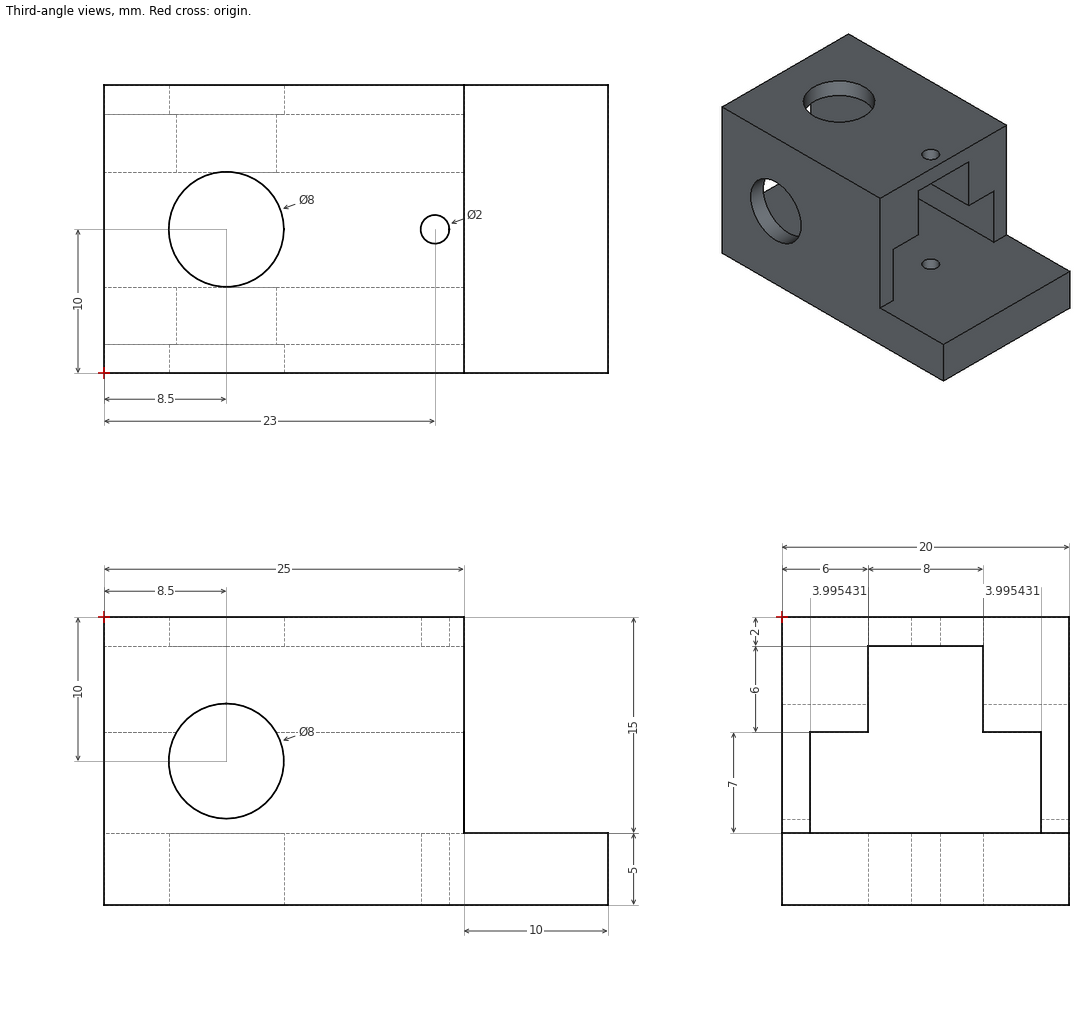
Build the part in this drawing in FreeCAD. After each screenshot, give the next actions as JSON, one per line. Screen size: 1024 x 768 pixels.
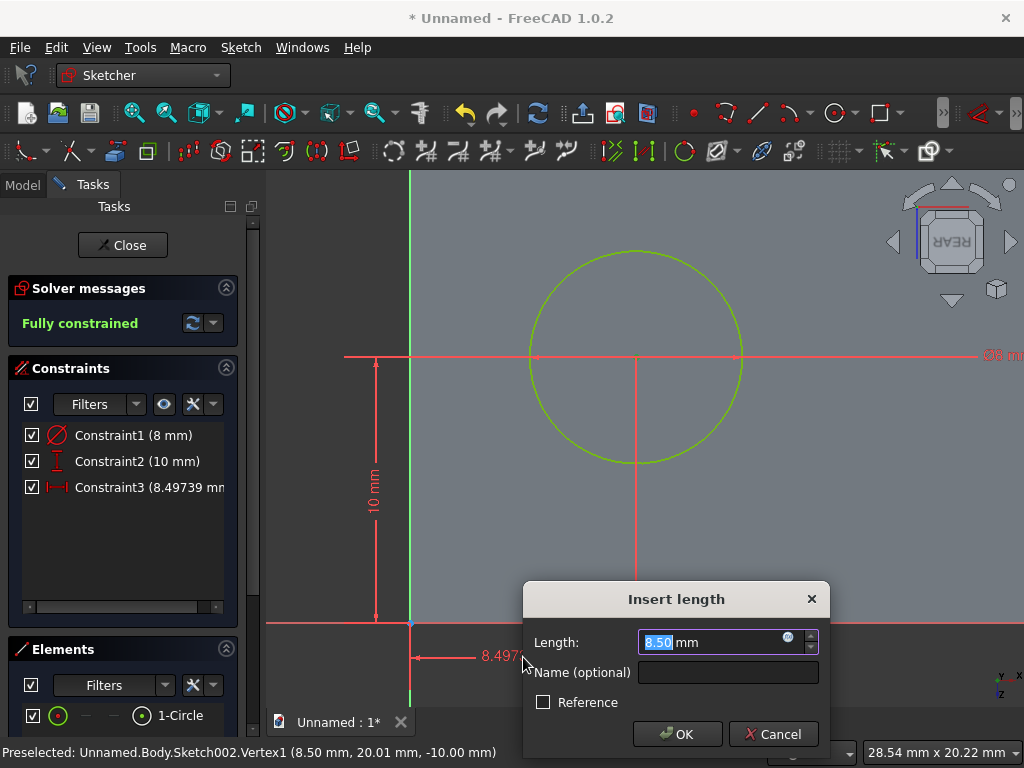
{"action": "type", "text": "8.5"}
{"action": "key", "text": "Return"}
{"action": "key", "text": "Escape"}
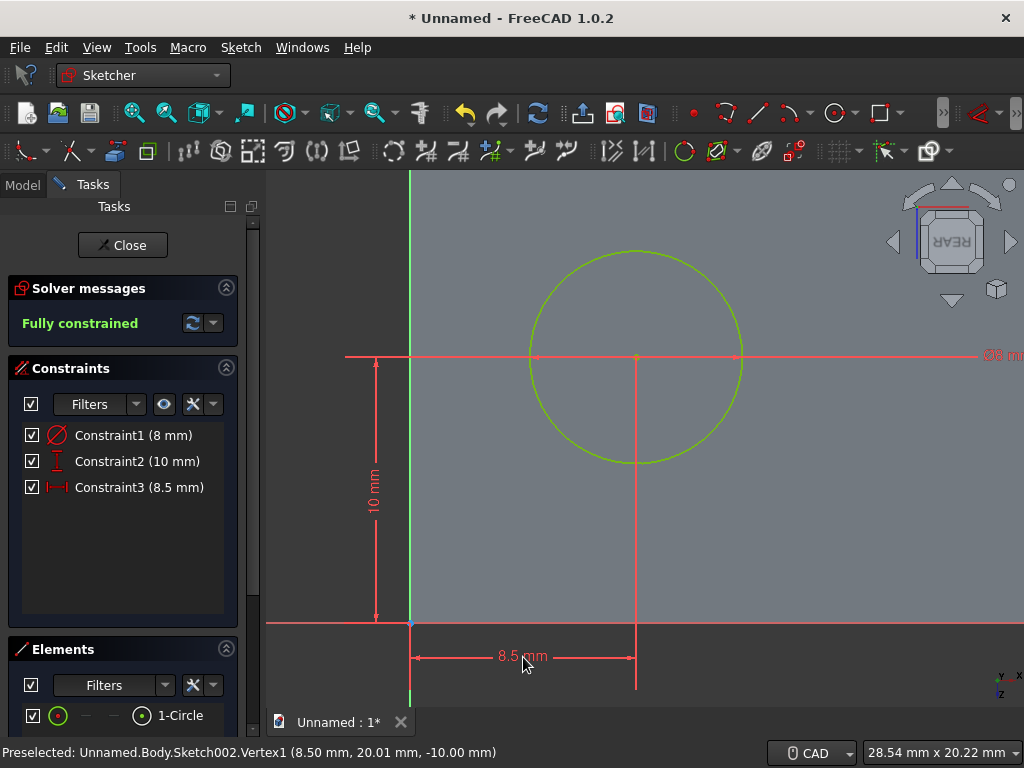
{"action": "left_click", "coordinate": [123, 245]}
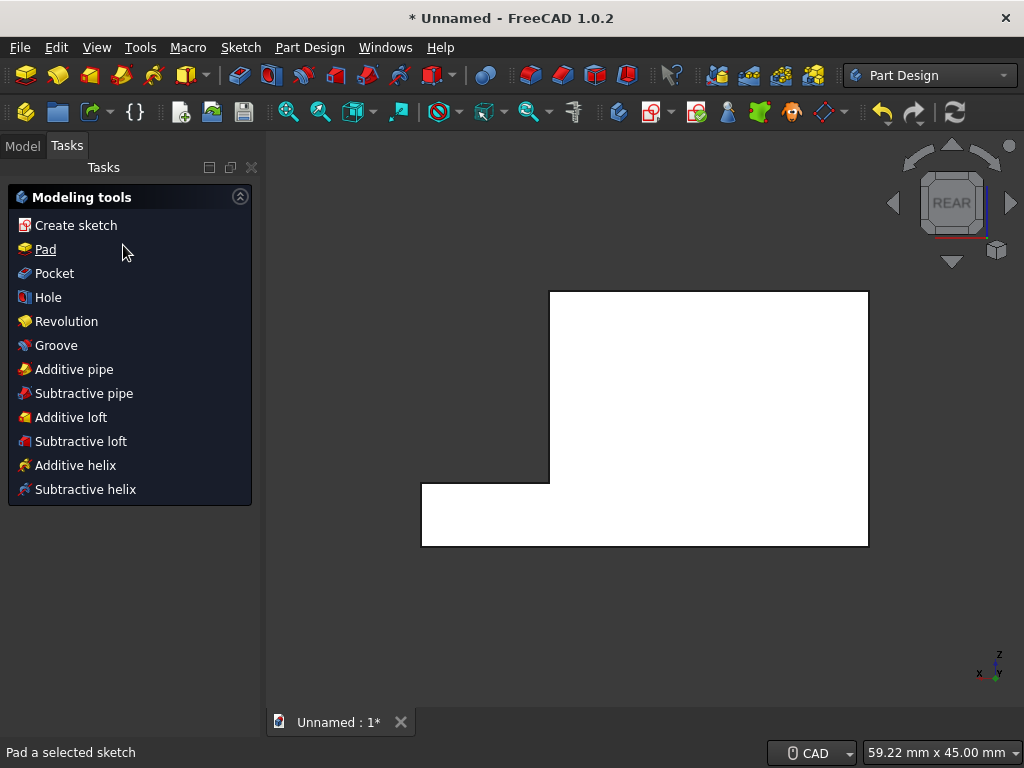
{"action": "left_click", "coordinate": [240, 76]}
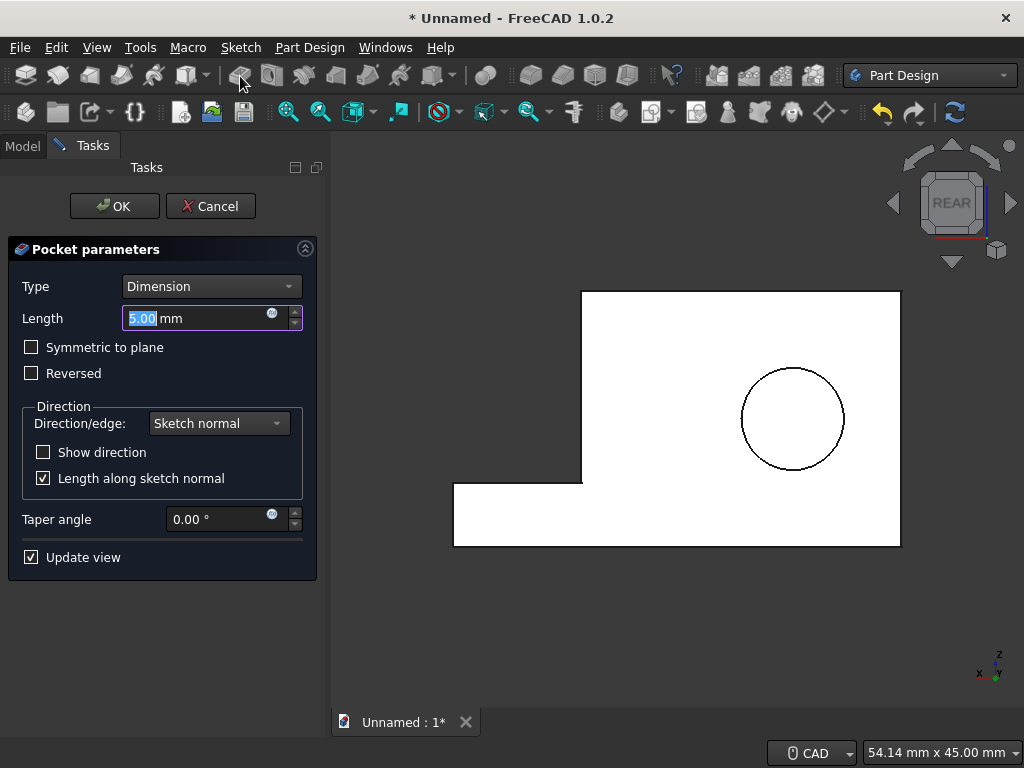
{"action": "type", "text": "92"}
{"action": "key", "text": "Tab"}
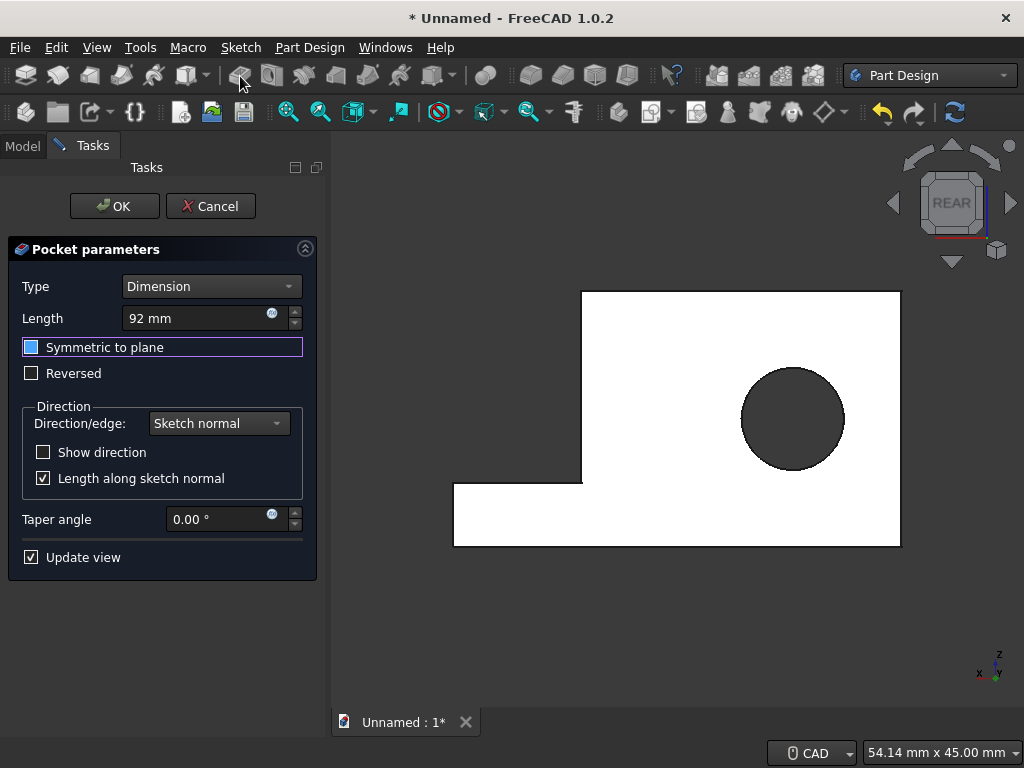
{"action": "left_click", "coordinate": [30, 347]}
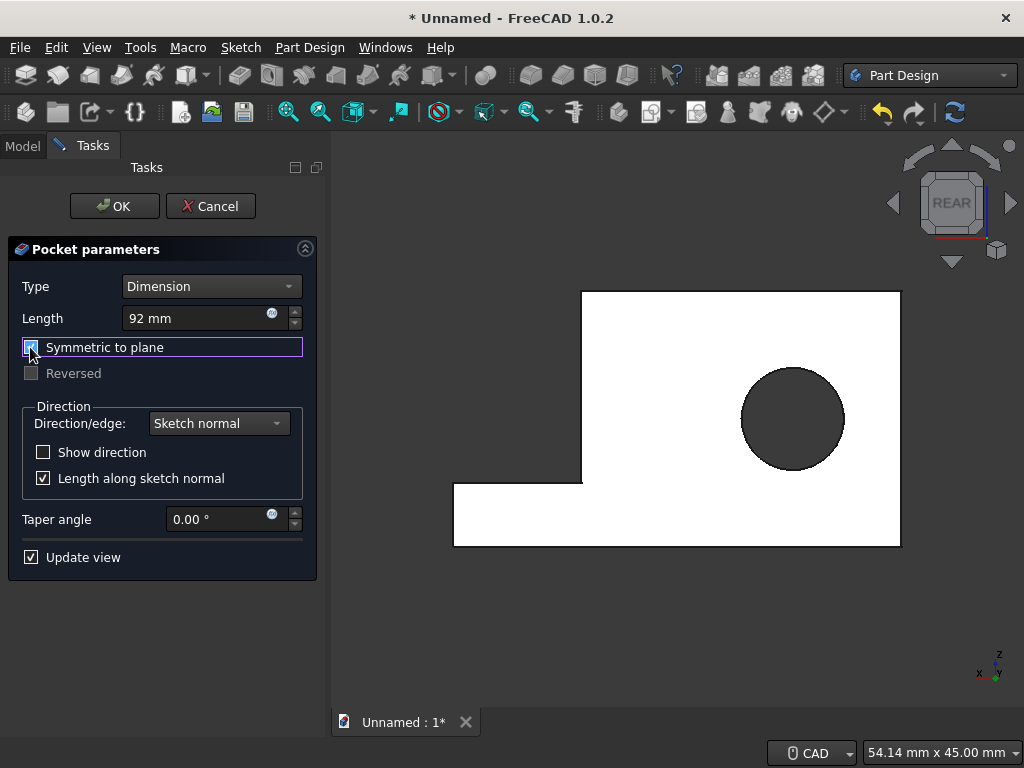
{"action": "left_click", "coordinate": [115, 206]}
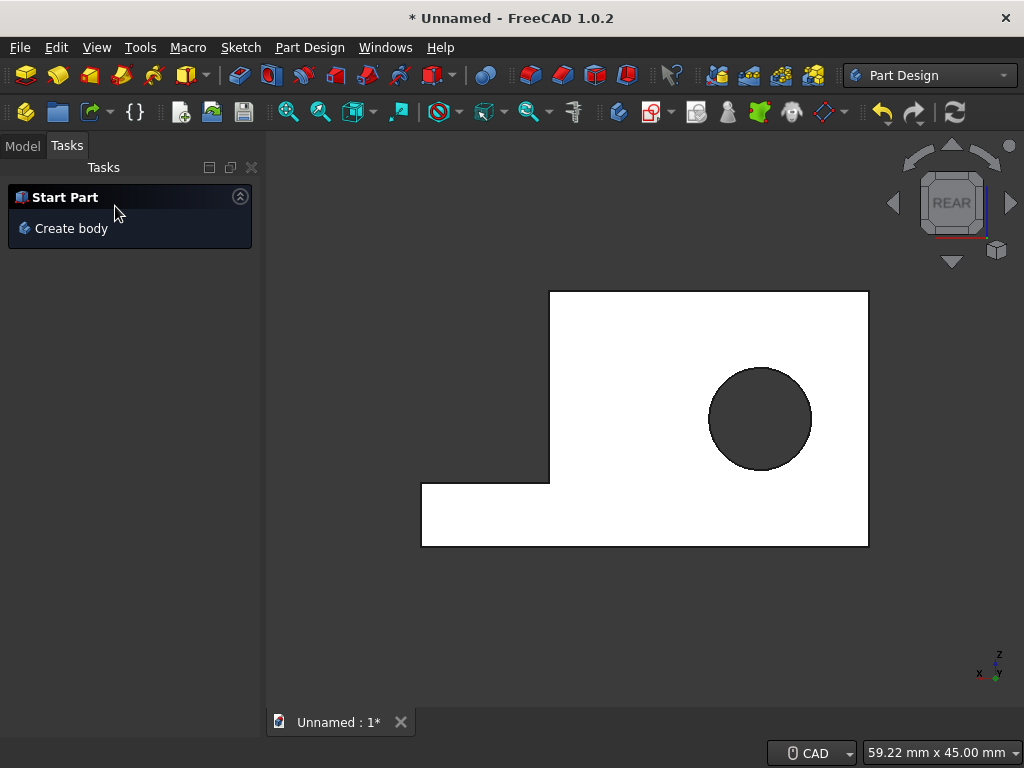
{"action": "key", "text": "0"}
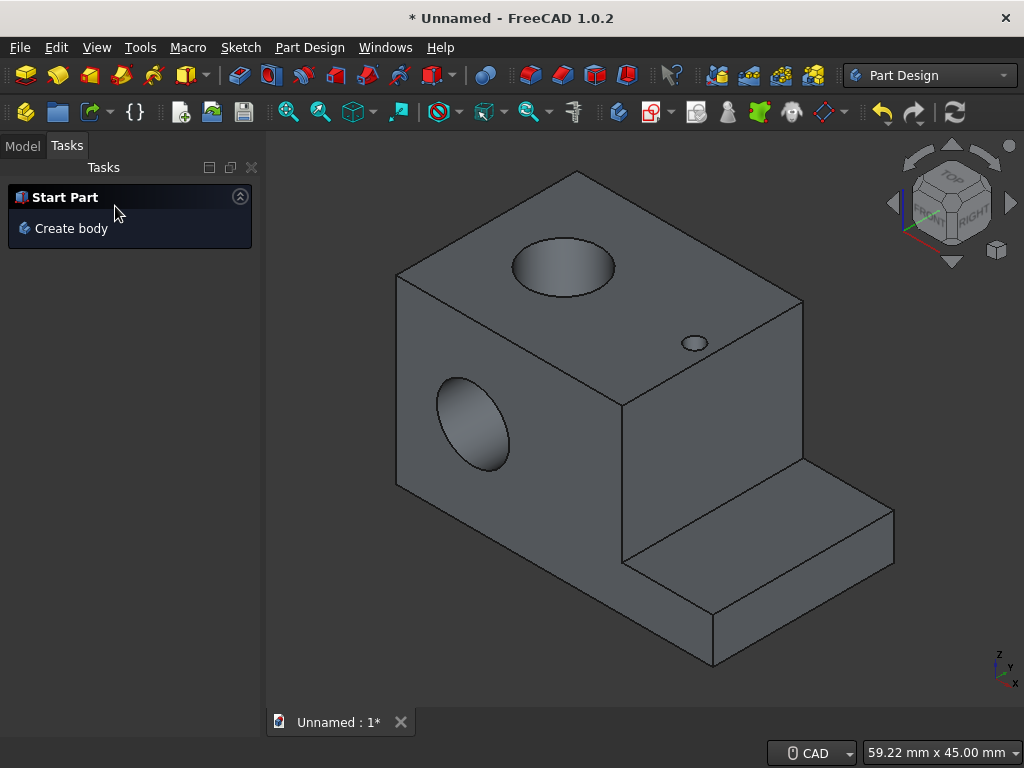
{"action": "left_click", "coordinate": [713, 431]}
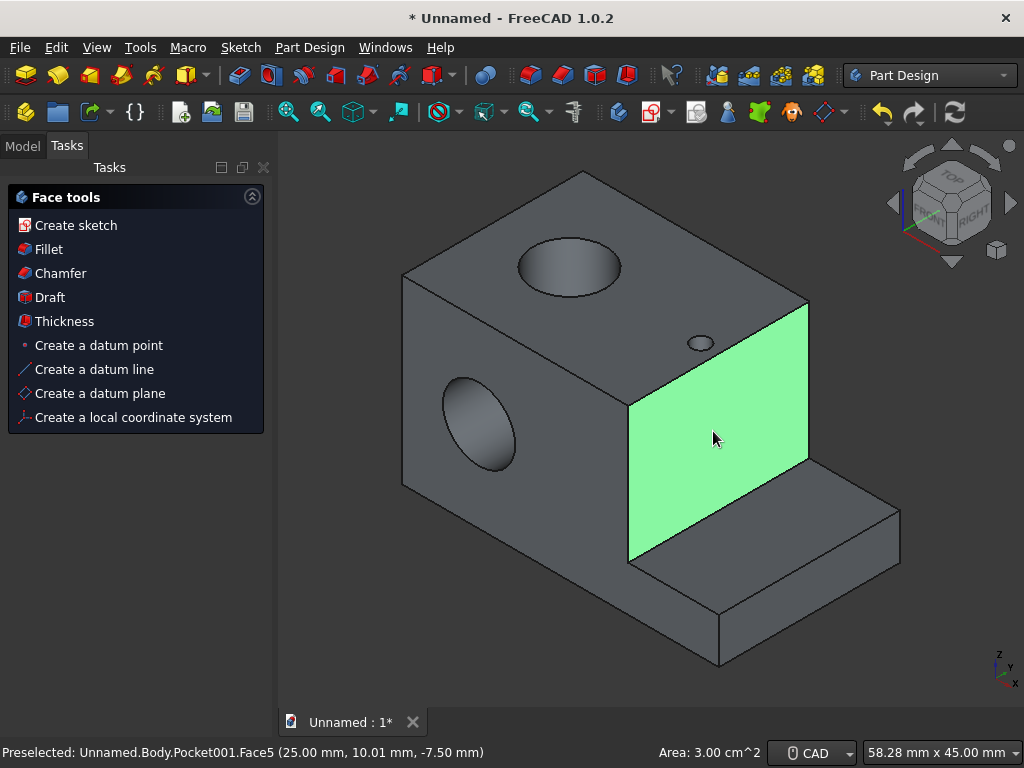
{"action": "left_click", "coordinate": [652, 112]}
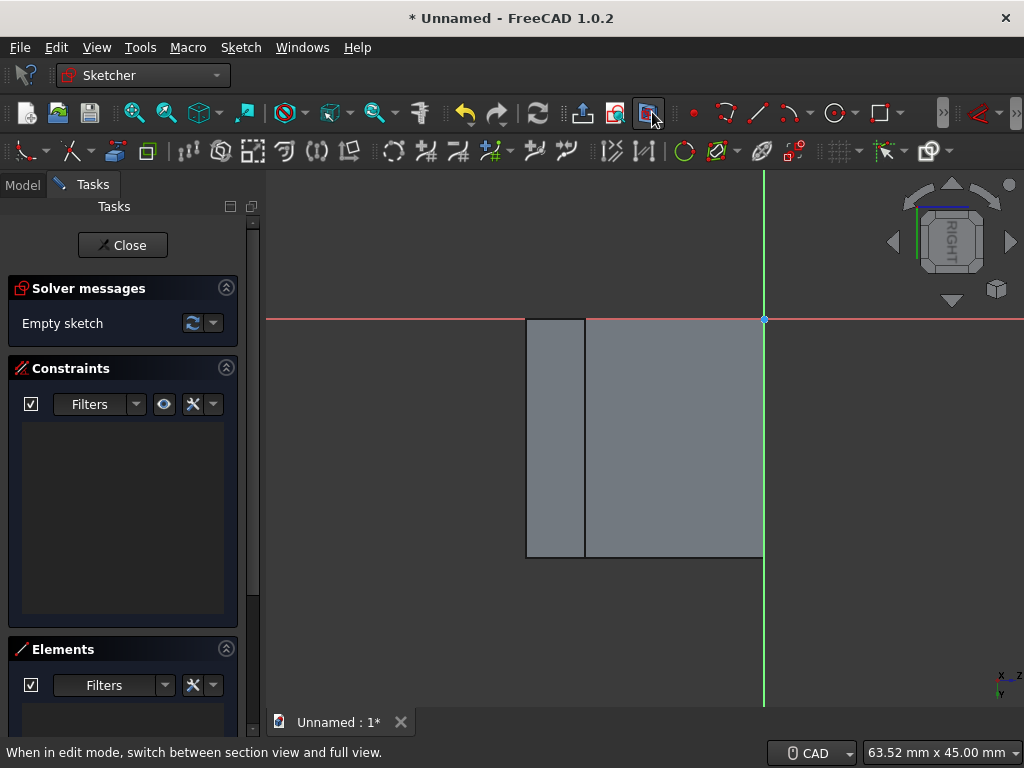
{"action": "scroll", "coordinate": [859, 402], "scroll_direction": "up", "scroll_amount": 2}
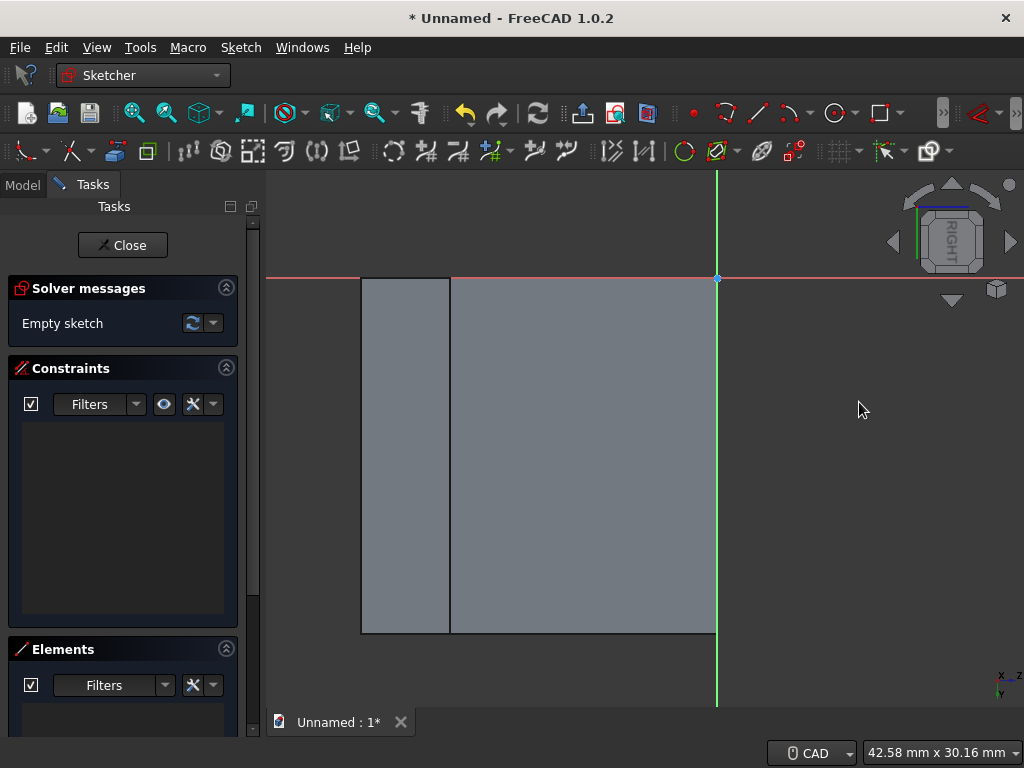
{"action": "left_click", "coordinate": [726, 114]}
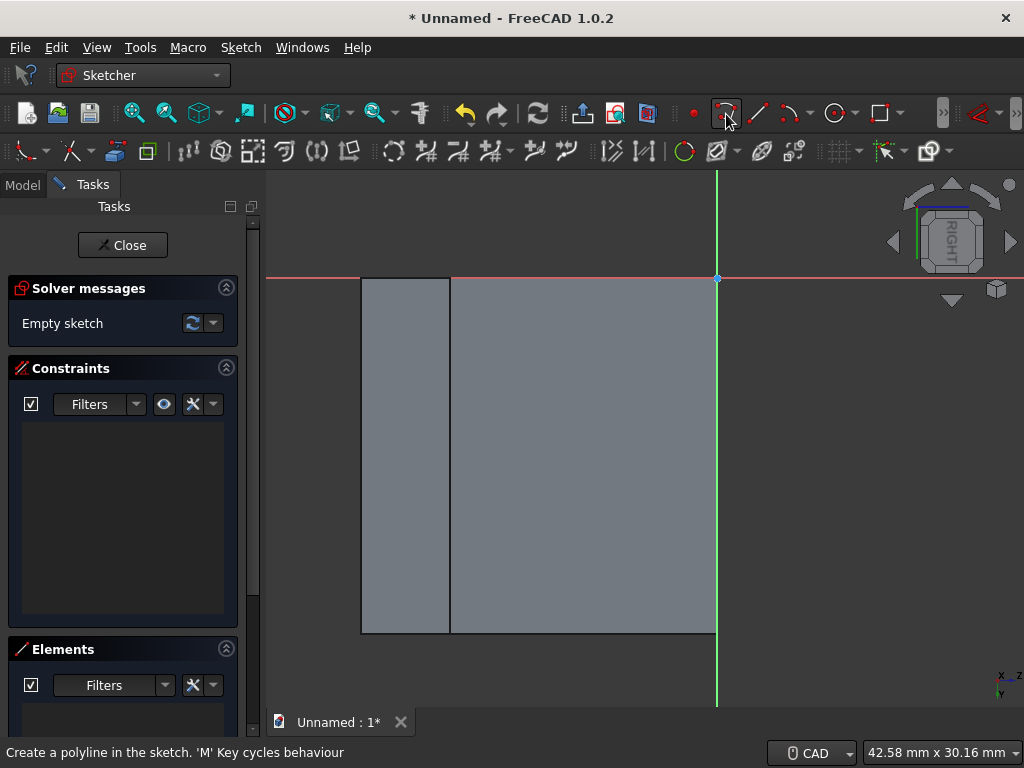
{"action": "left_click", "coordinate": [682, 385]}
{"action": "left_click", "coordinate": [575, 385]}
{"action": "left_click", "coordinate": [575, 314]}
{"action": "left_click", "coordinate": [450, 314]}
{"action": "left_click", "coordinate": [450, 599]}
{"action": "left_click", "coordinate": [575, 599]}
{"action": "left_click", "coordinate": [575, 527]}
{"action": "left_click", "coordinate": [682, 527]}
{"action": "left_click", "coordinate": [682, 386]}
{"action": "key", "text": "Escape"}
{"action": "key", "text": "Escape"}